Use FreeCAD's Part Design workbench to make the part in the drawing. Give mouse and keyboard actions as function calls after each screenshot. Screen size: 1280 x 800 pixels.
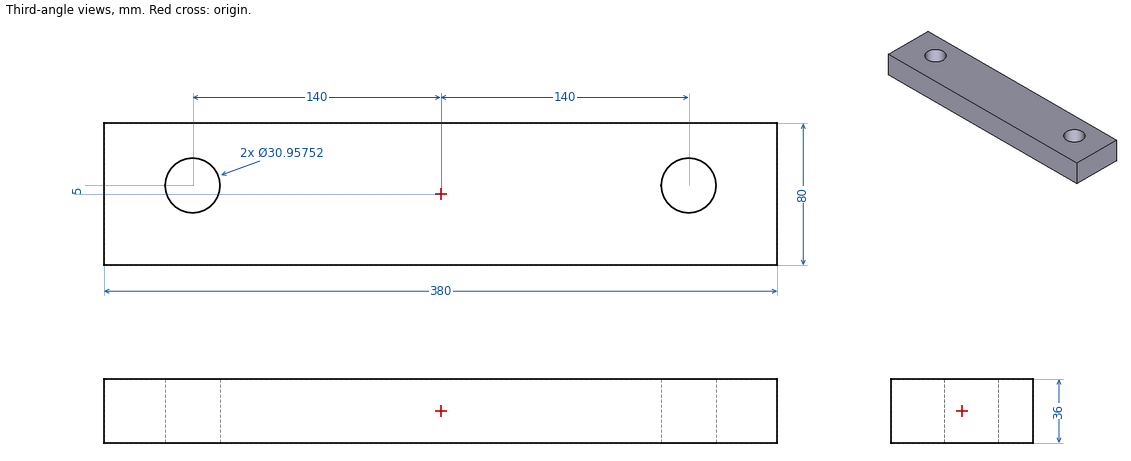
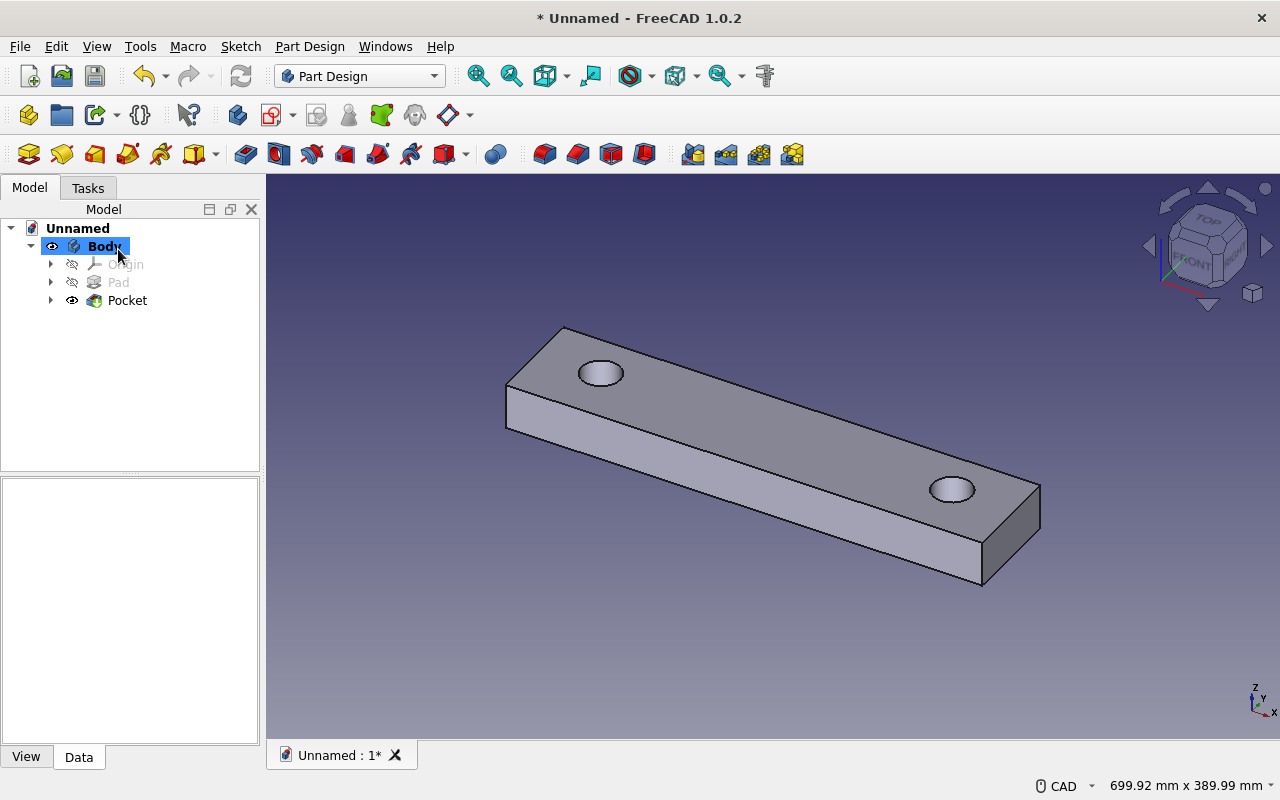
key(0)